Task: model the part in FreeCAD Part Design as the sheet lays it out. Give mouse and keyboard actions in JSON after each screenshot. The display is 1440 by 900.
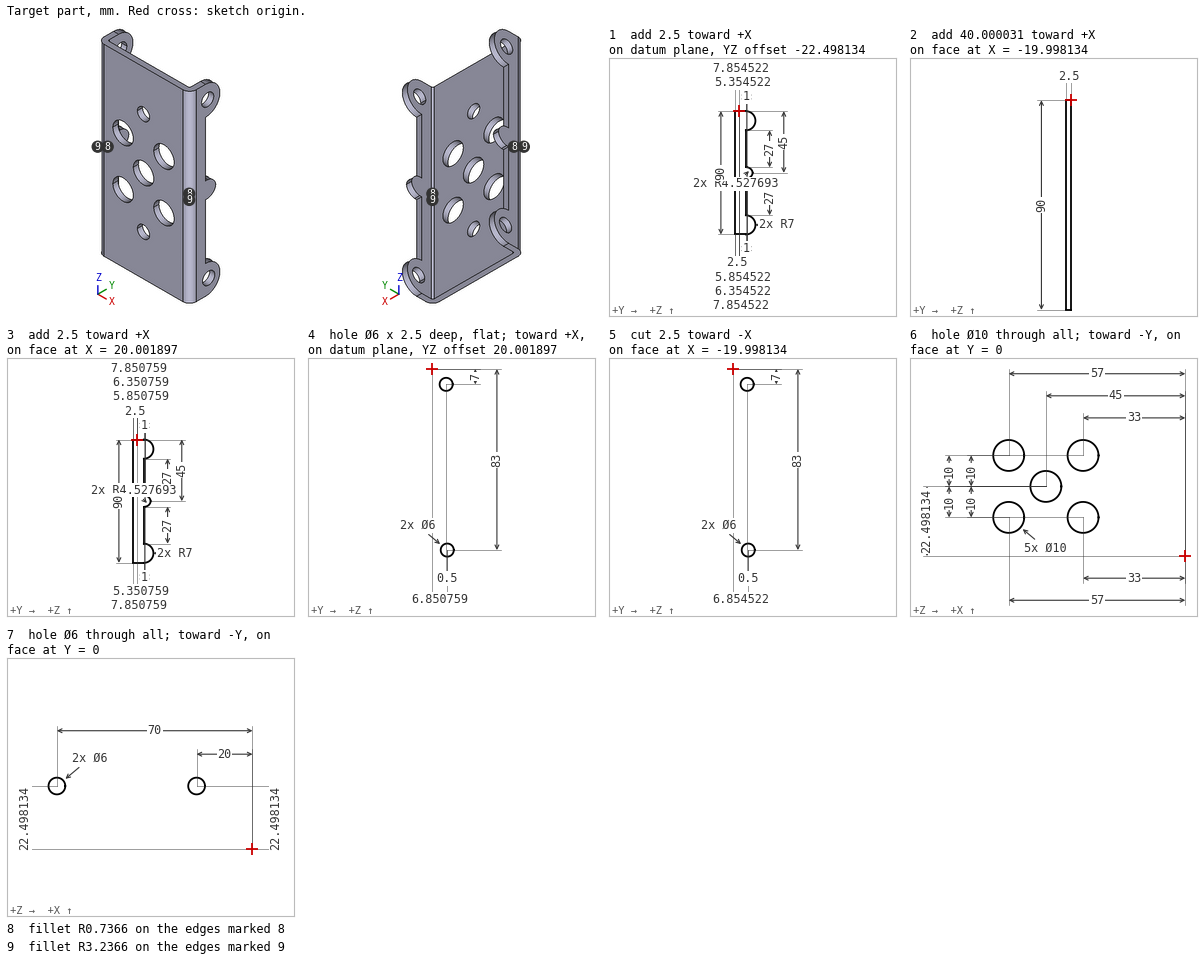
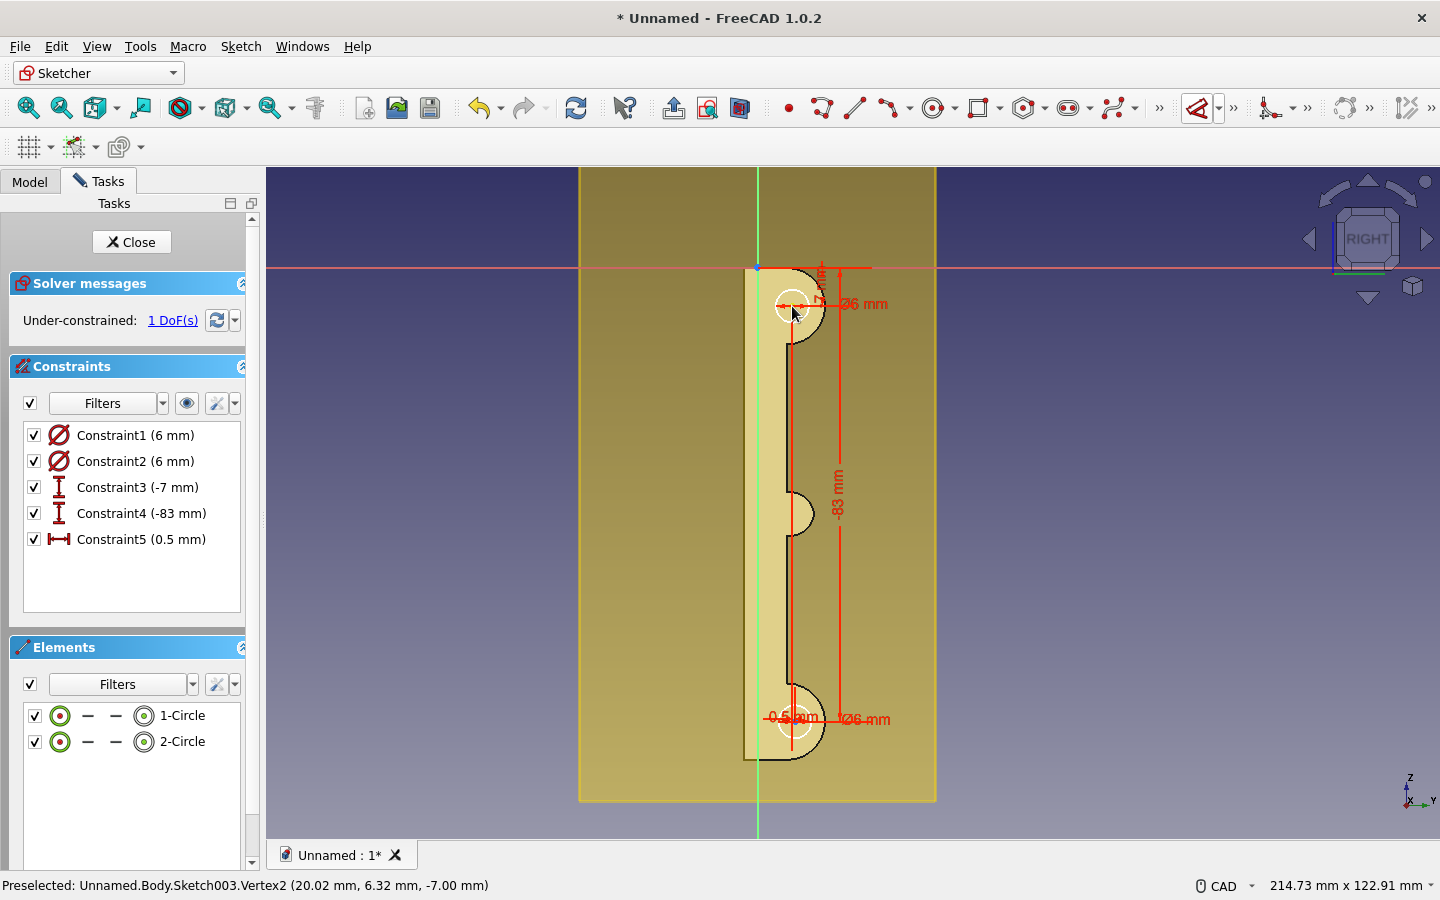
{"action": "left_click", "coordinate": [795, 722]}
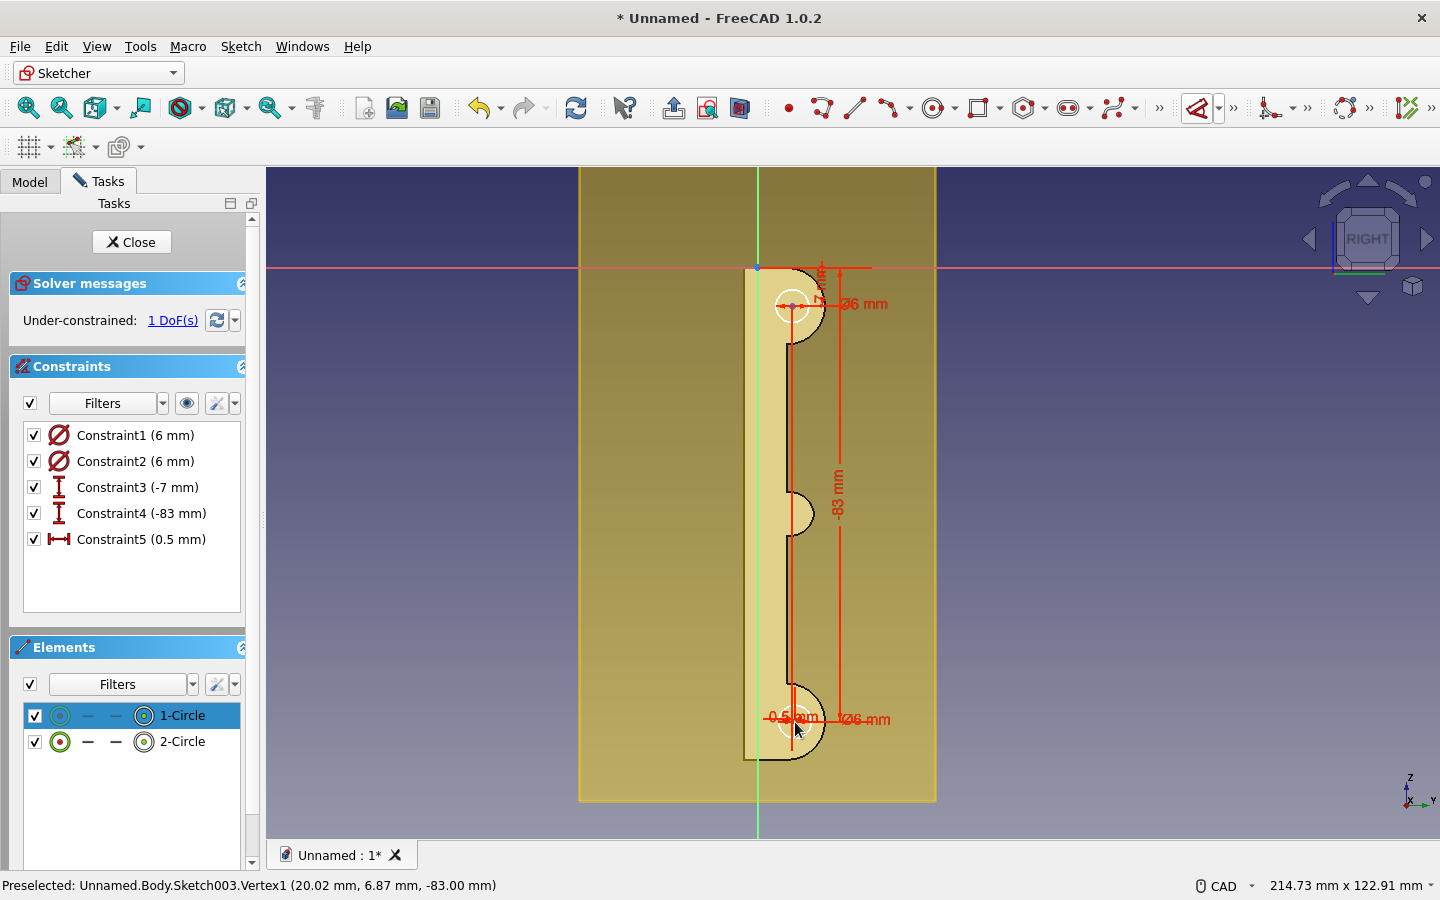
{"action": "left_click", "coordinate": [1218, 108]}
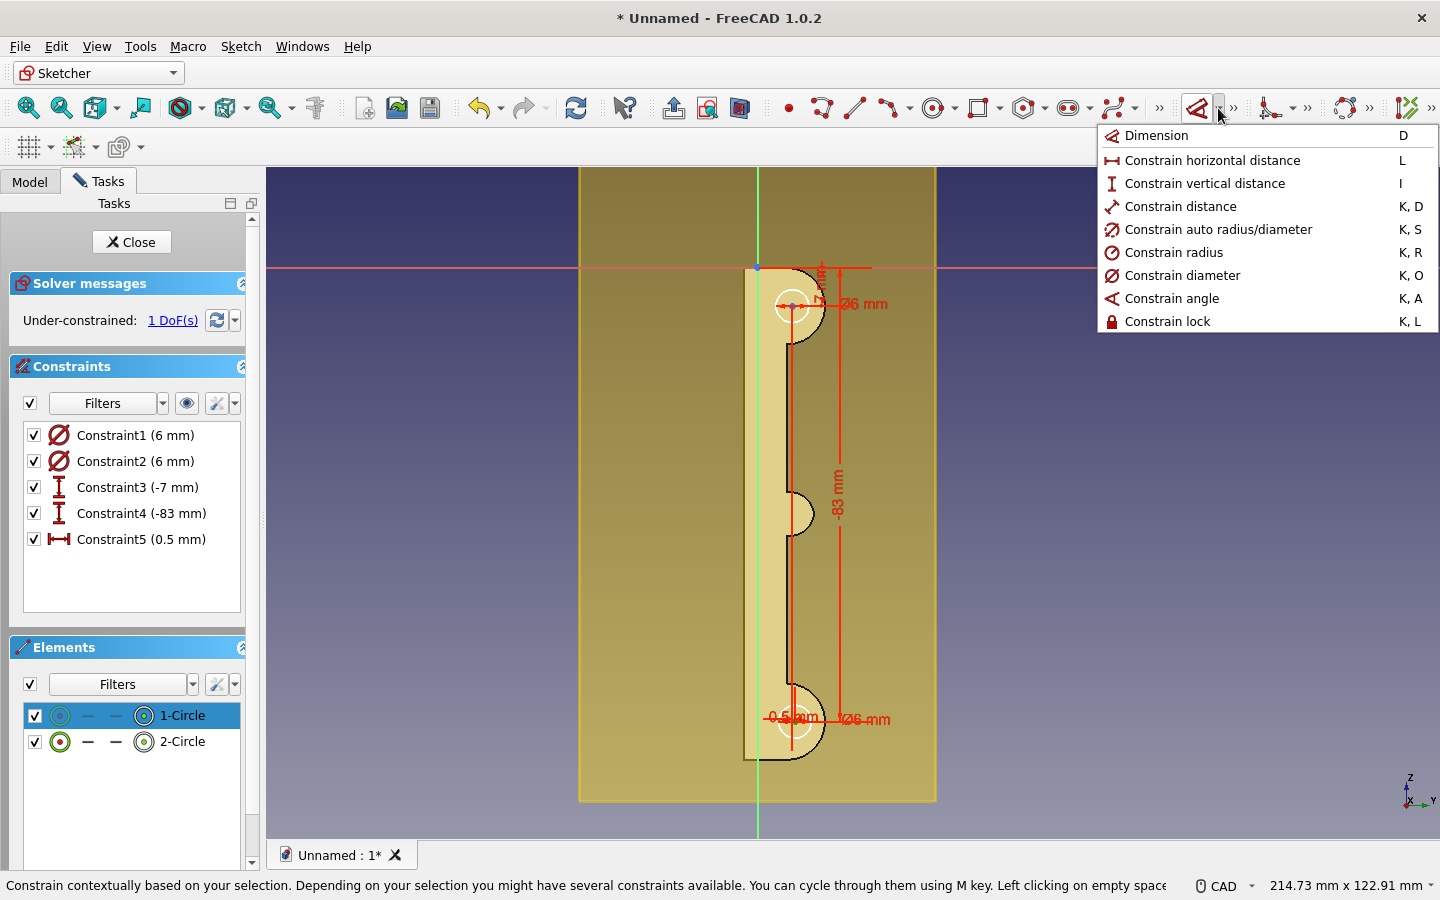
{"action": "left_click", "coordinate": [1268, 160]}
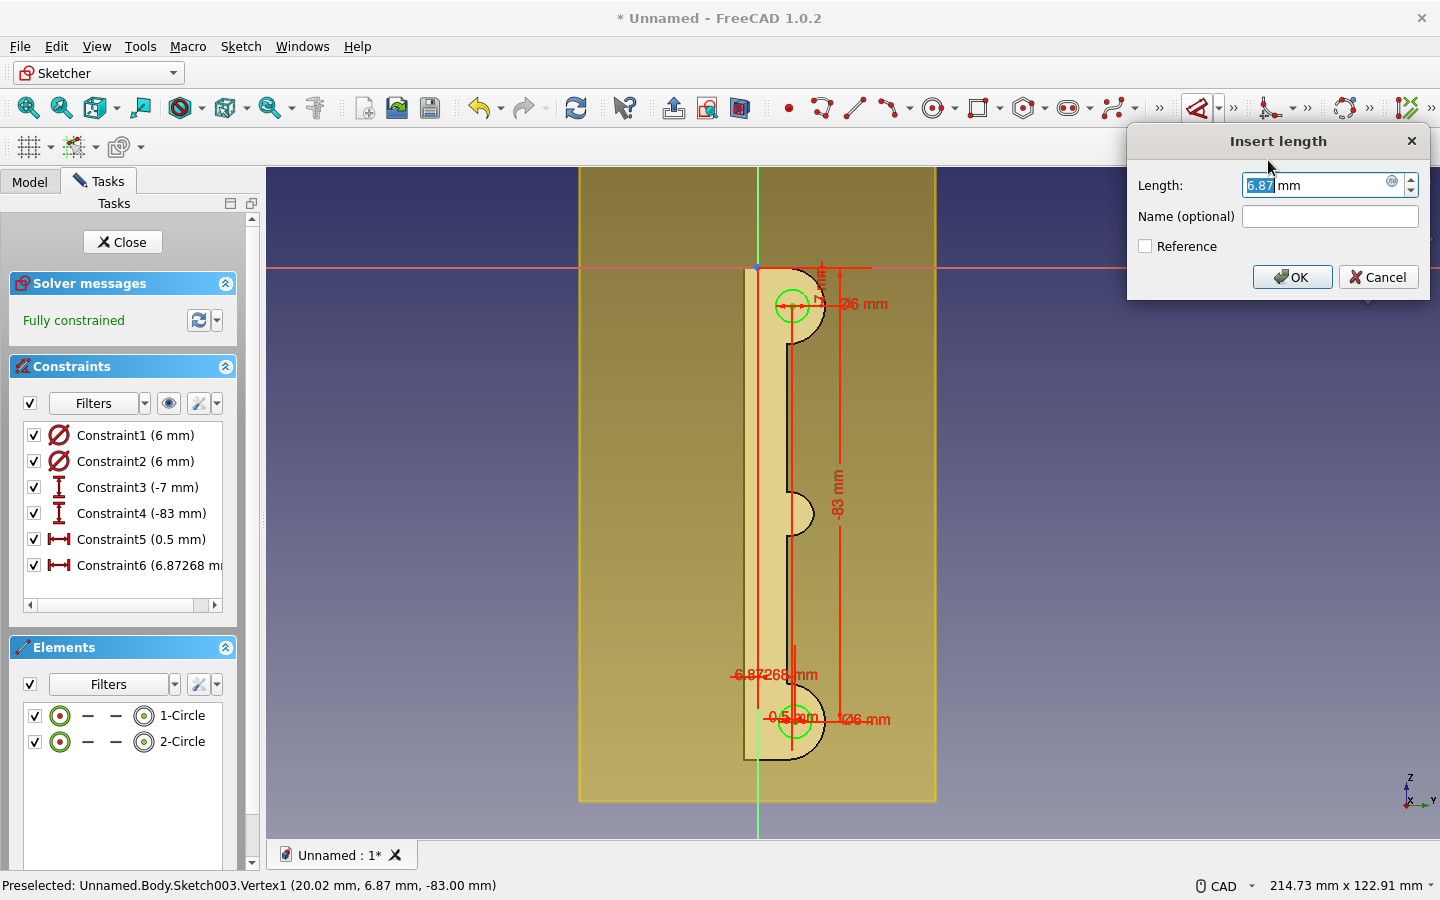
{"action": "type", "text": "6.850759"}
{"action": "key", "text": "Return"}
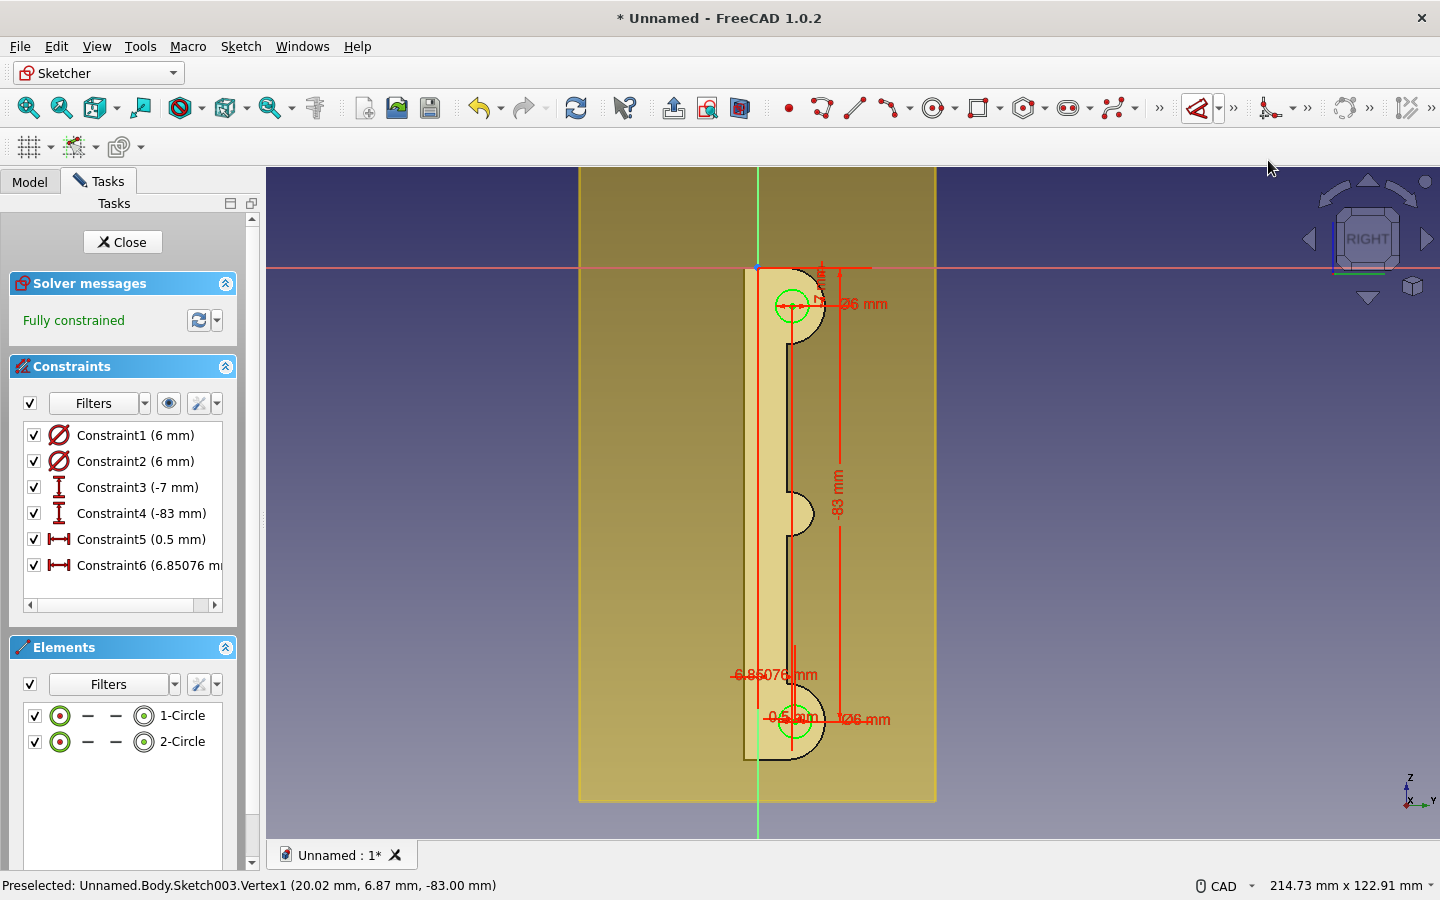
{"action": "left_click", "coordinate": [123, 242]}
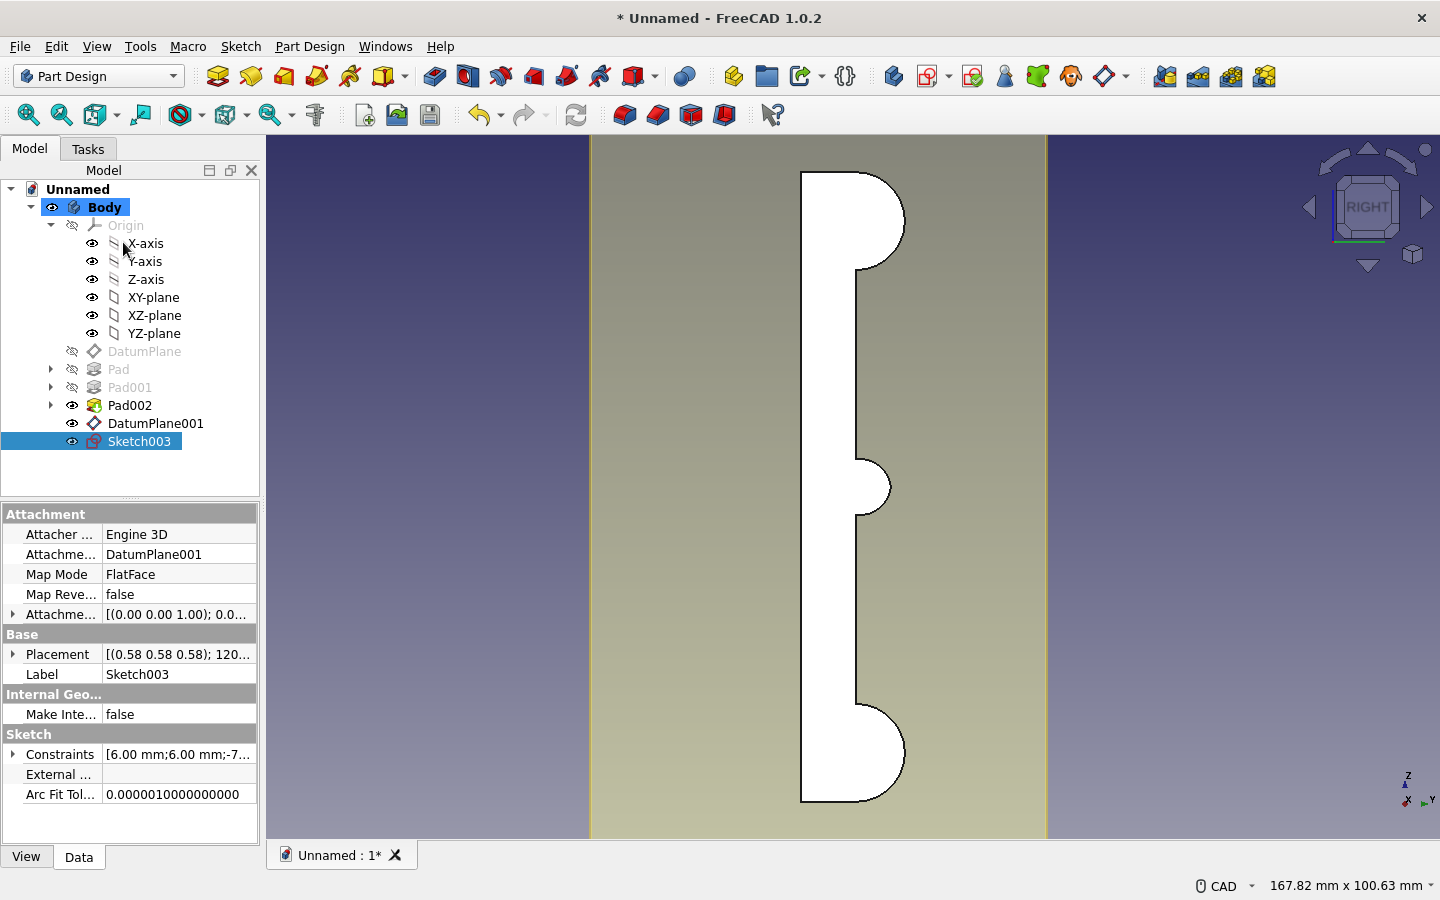
{"action": "left_click", "coordinate": [468, 76]}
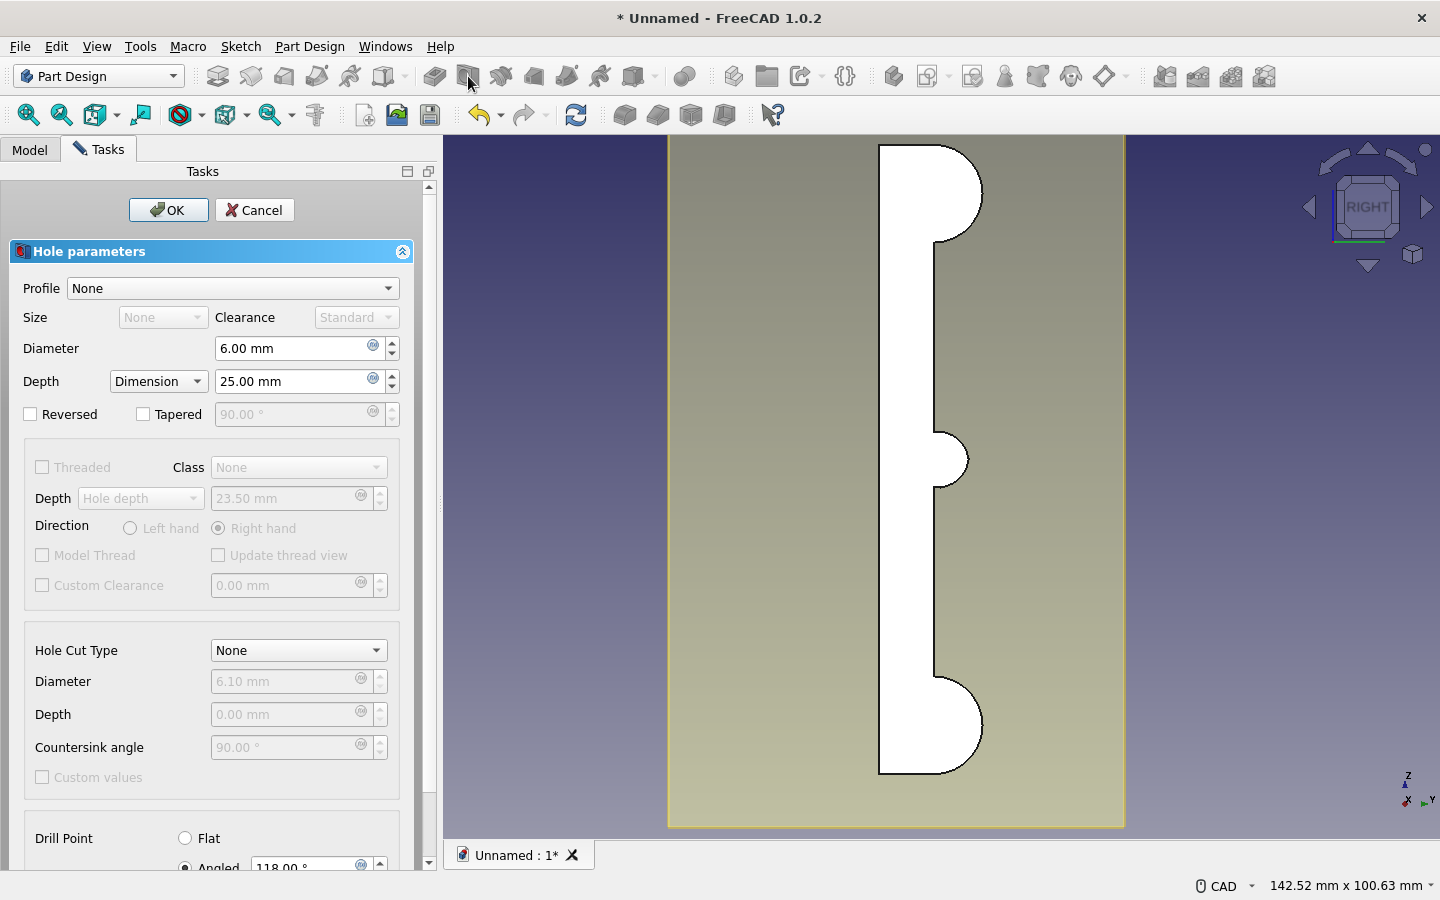
{"action": "triple_click", "coordinate": [300, 348]}